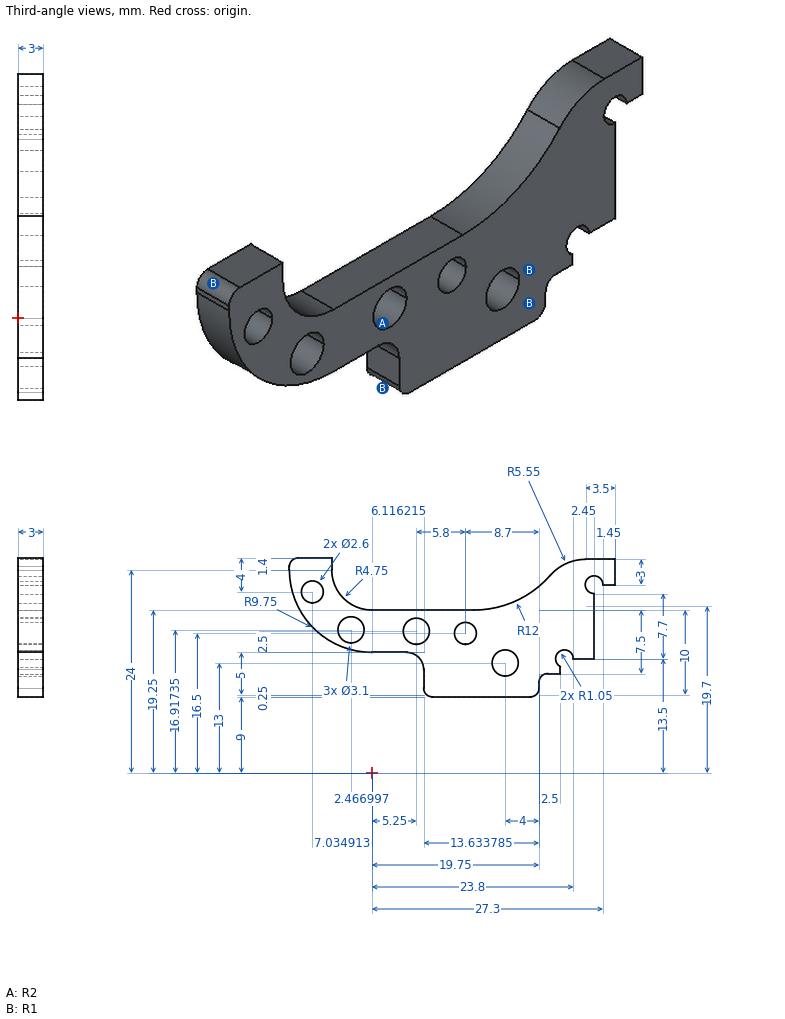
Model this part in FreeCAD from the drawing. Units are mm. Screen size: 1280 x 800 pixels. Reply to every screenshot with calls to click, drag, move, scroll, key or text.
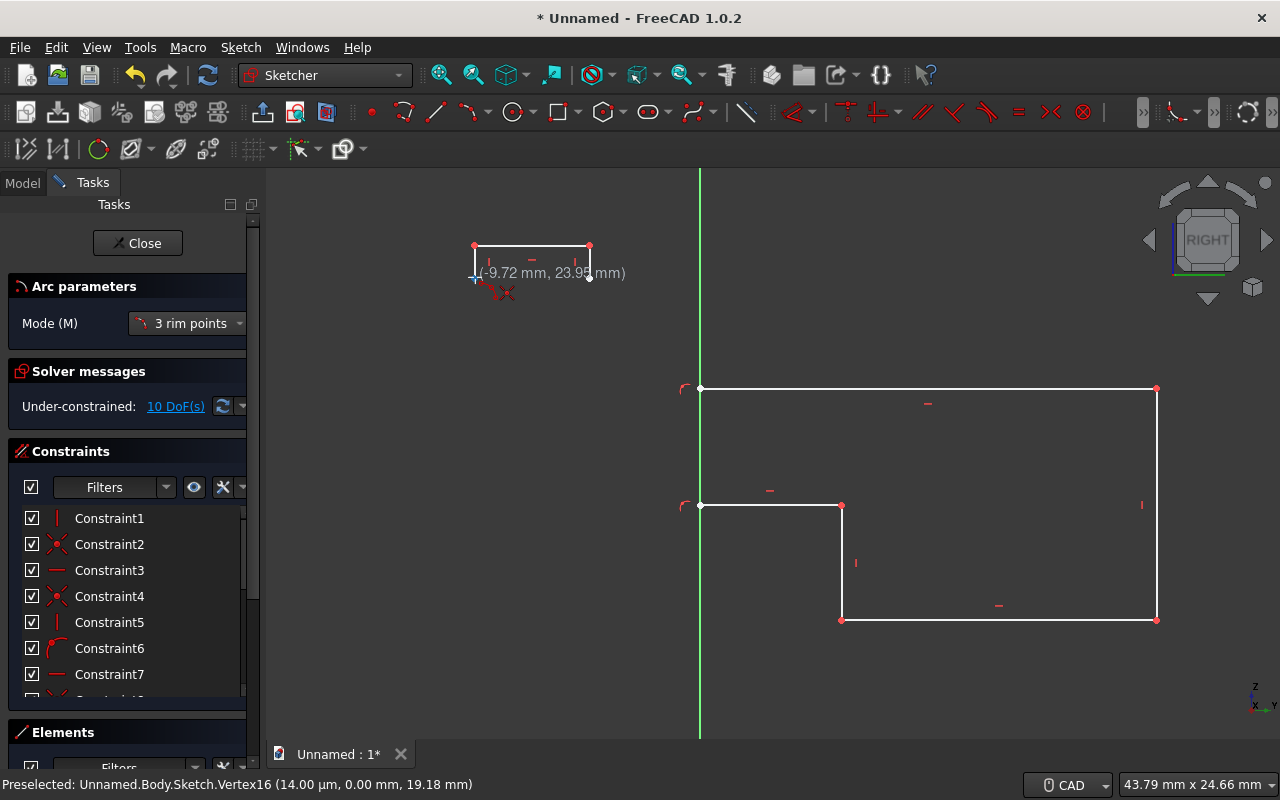
click(475, 278)
click(700, 505)
click(540, 437)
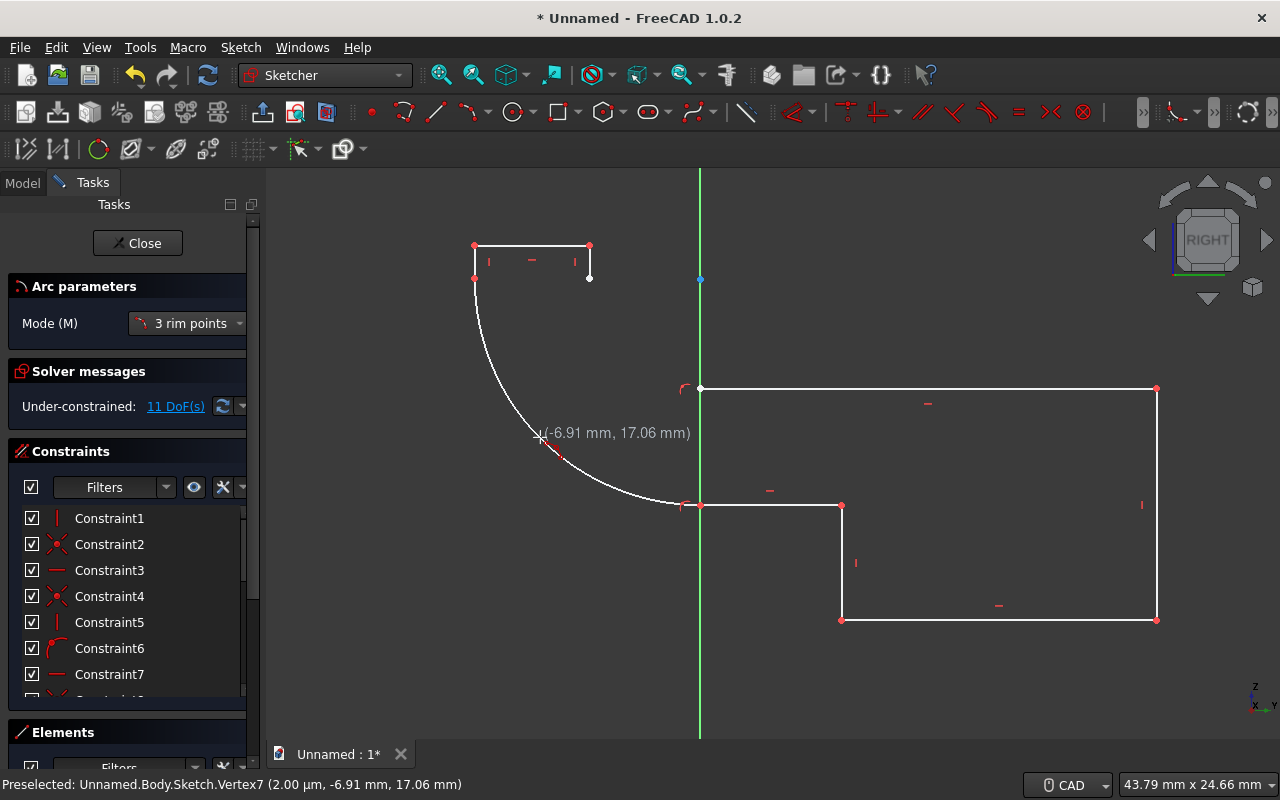
click(700, 389)
click(590, 278)
click(622, 355)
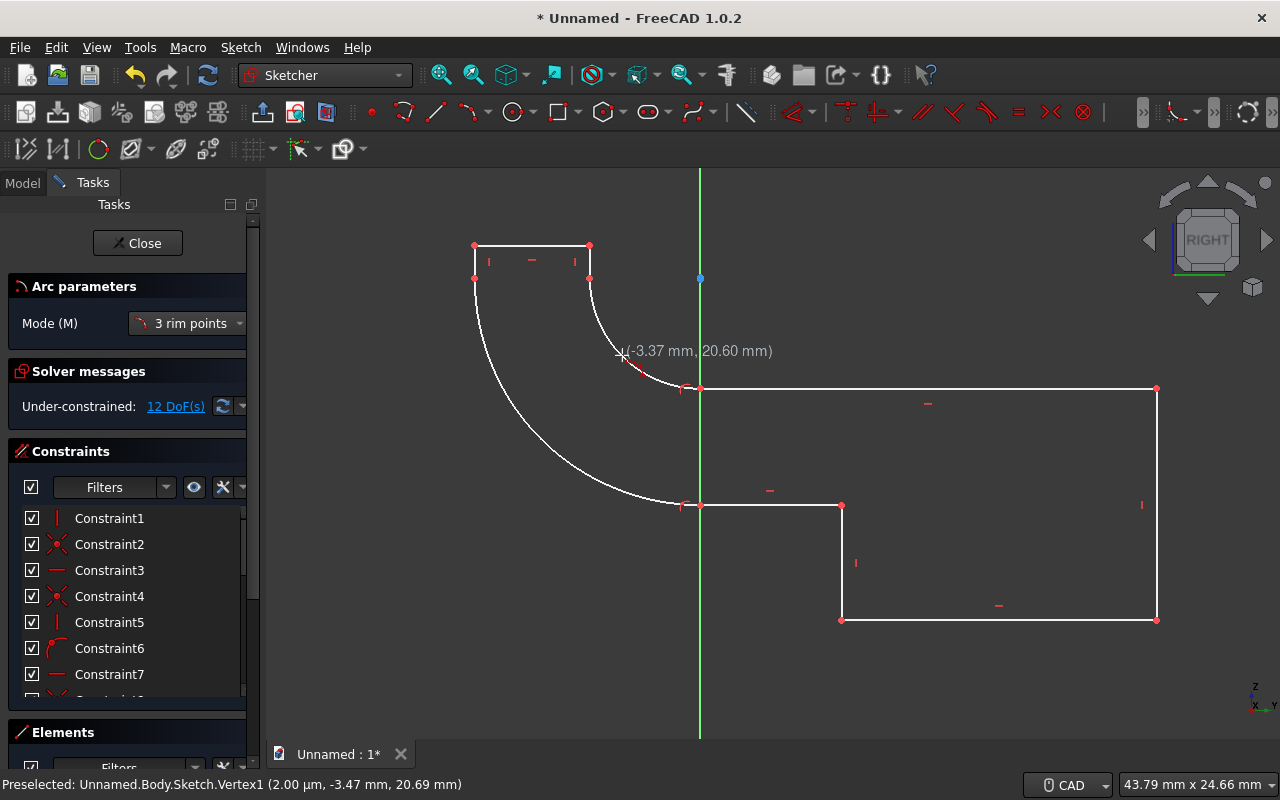
key(g)
key(c)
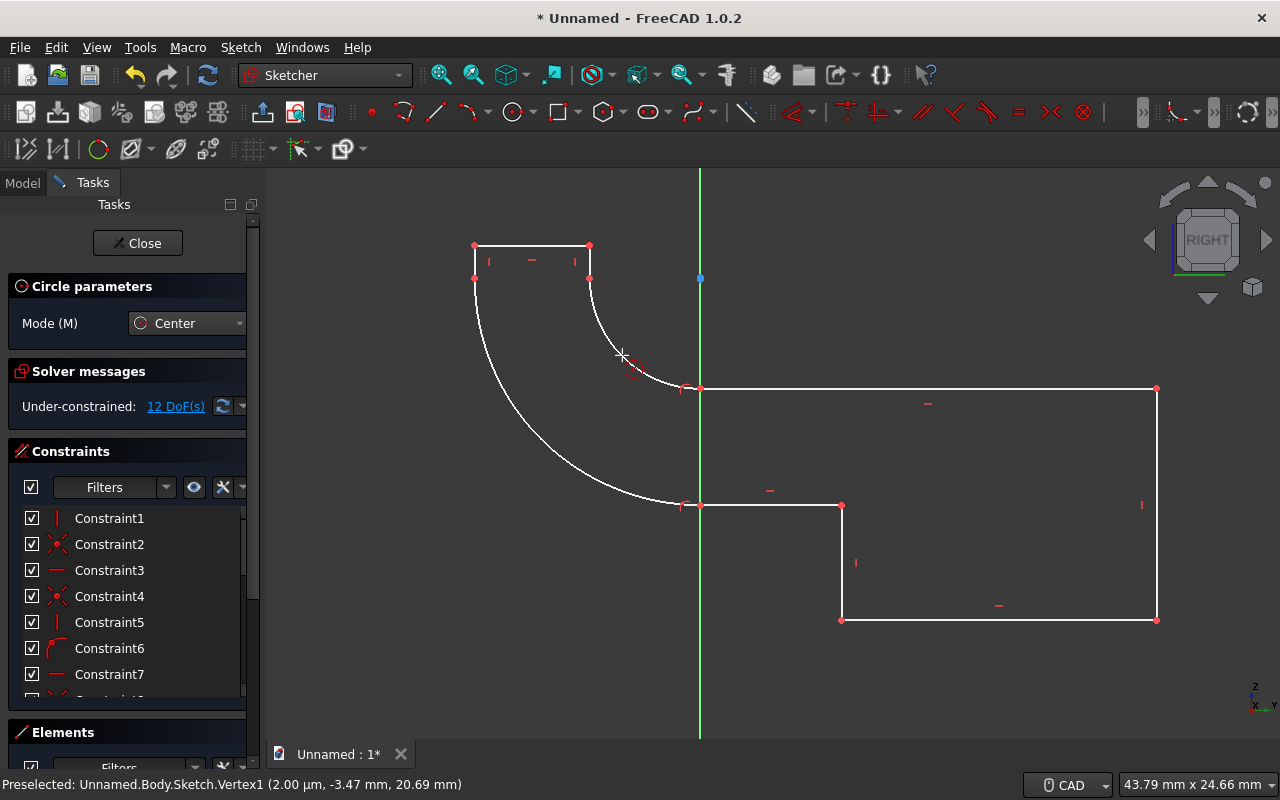
click(537, 337)
click(558, 316)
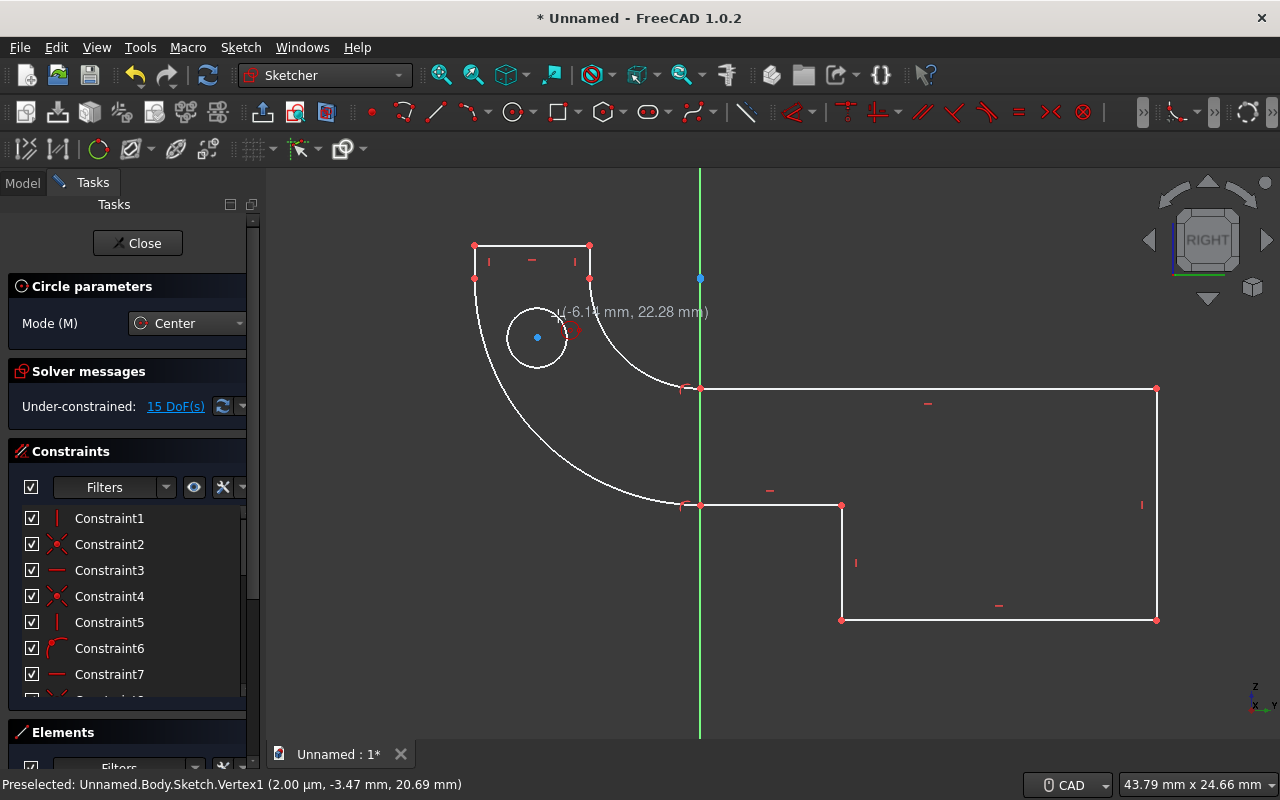
click(643, 441)
click(668, 416)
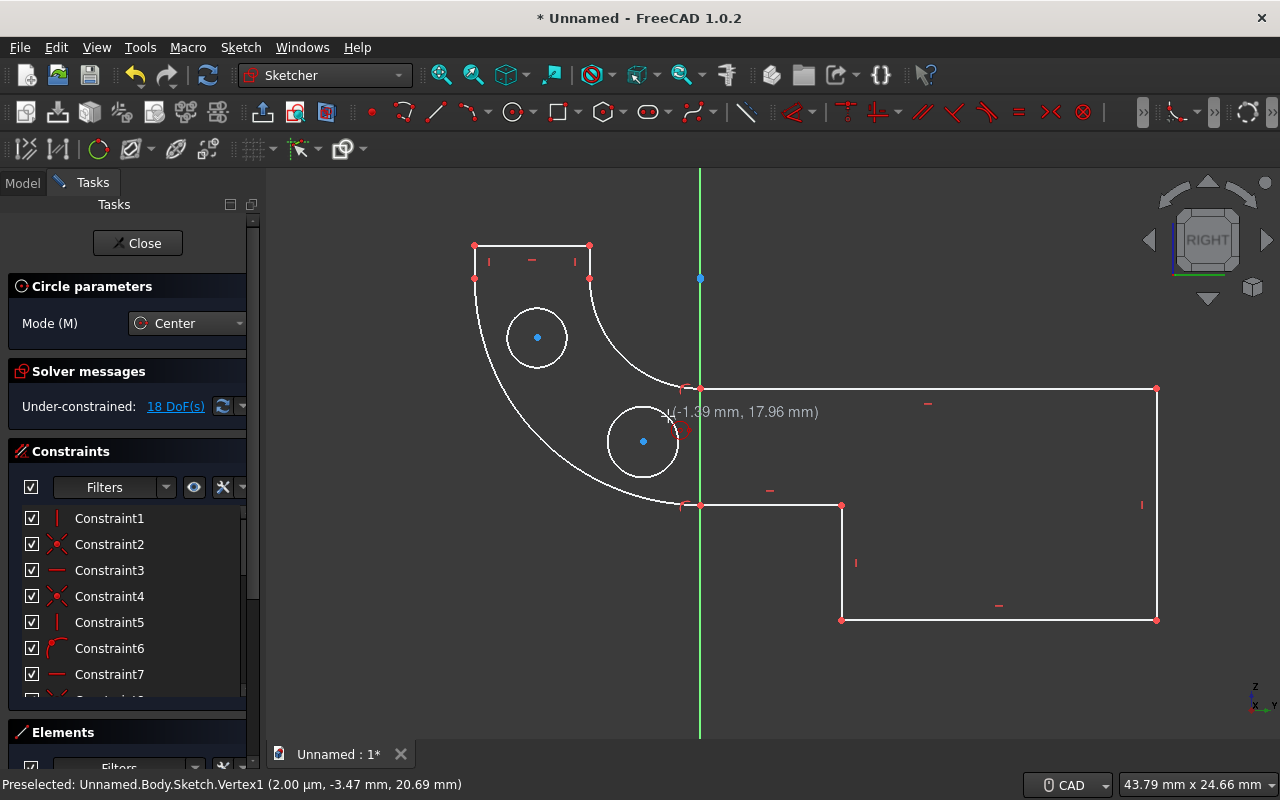
click(822, 445)
click(847, 420)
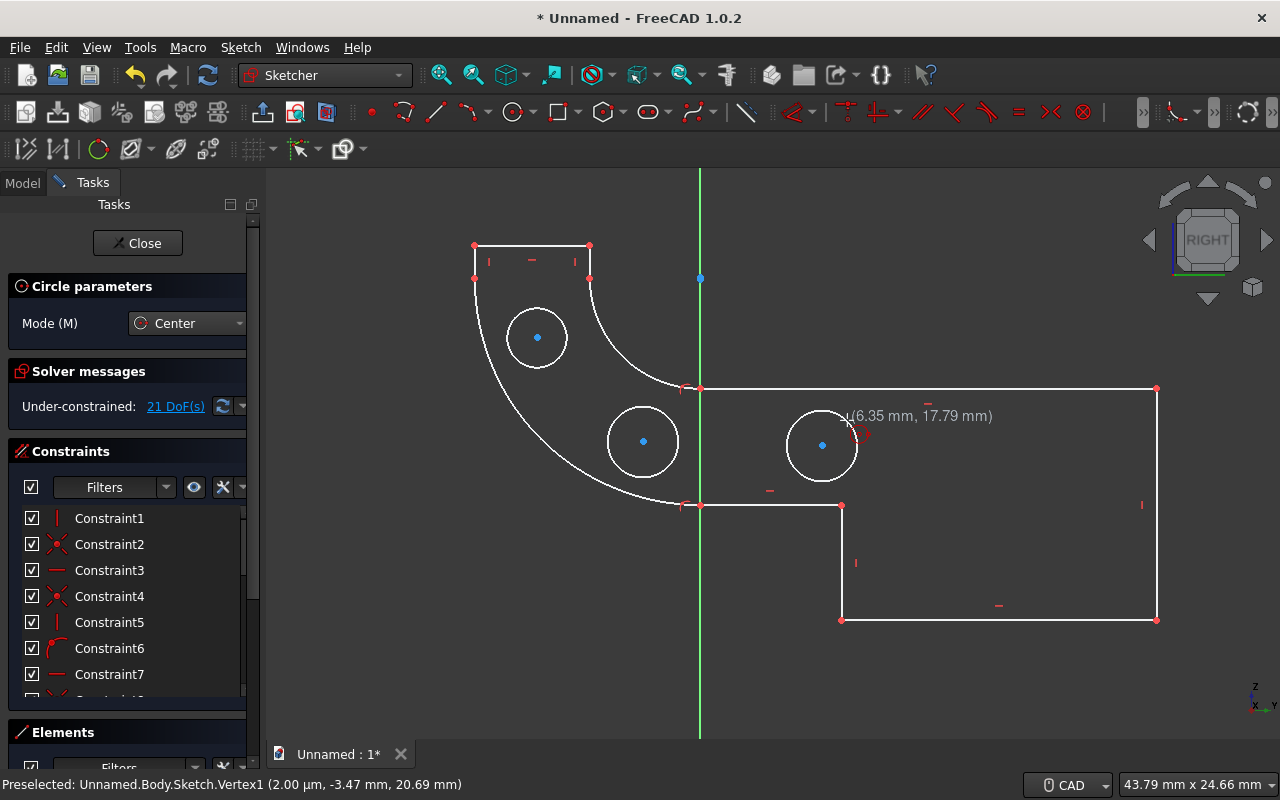
click(956, 451)
click(977, 430)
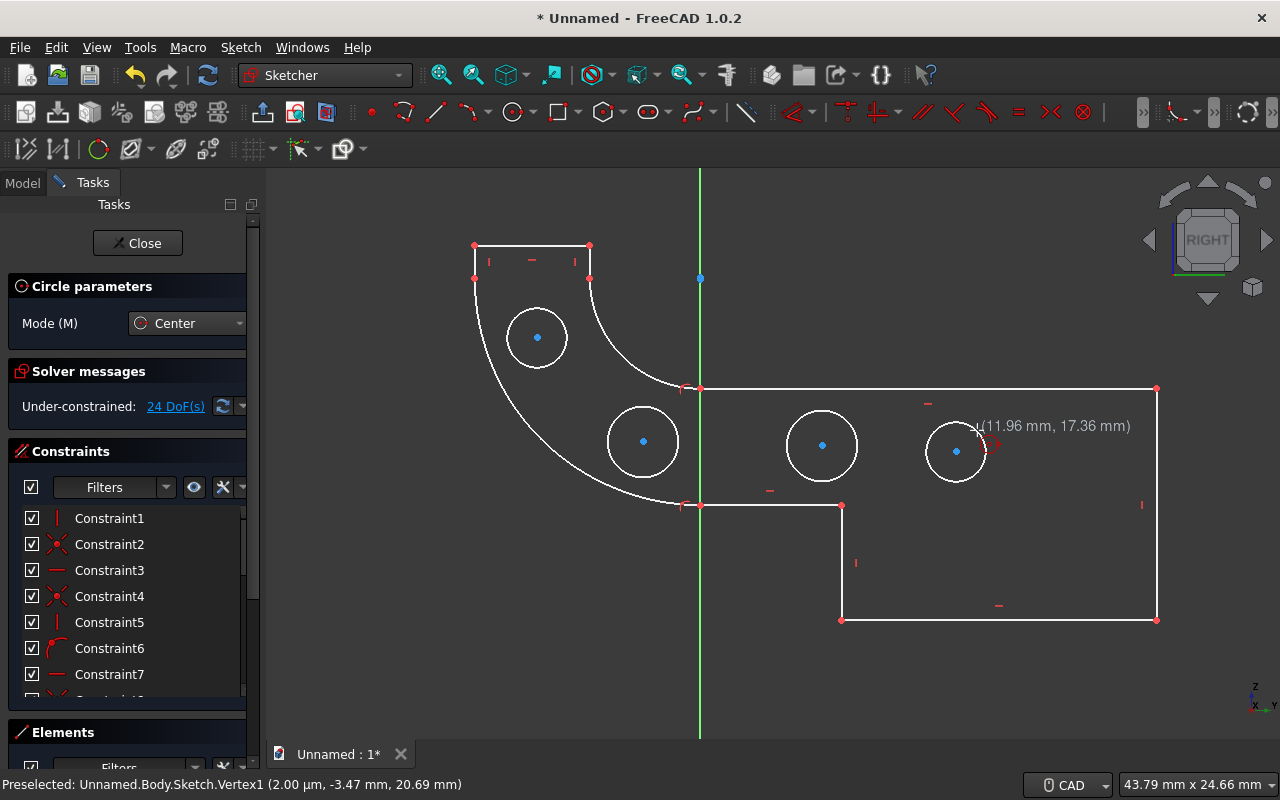
click(1065, 532)
click(1090, 507)
key(Escape)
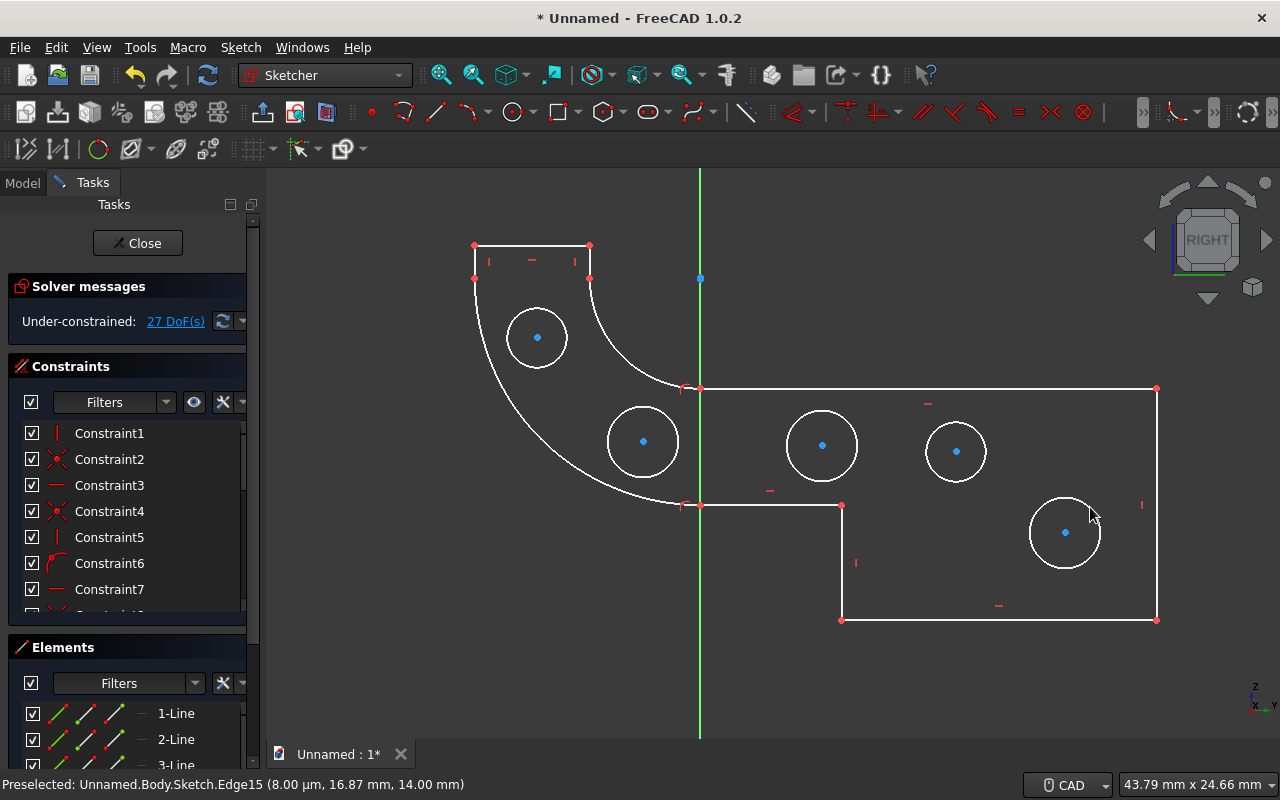
scroll(590, 269, up, 2)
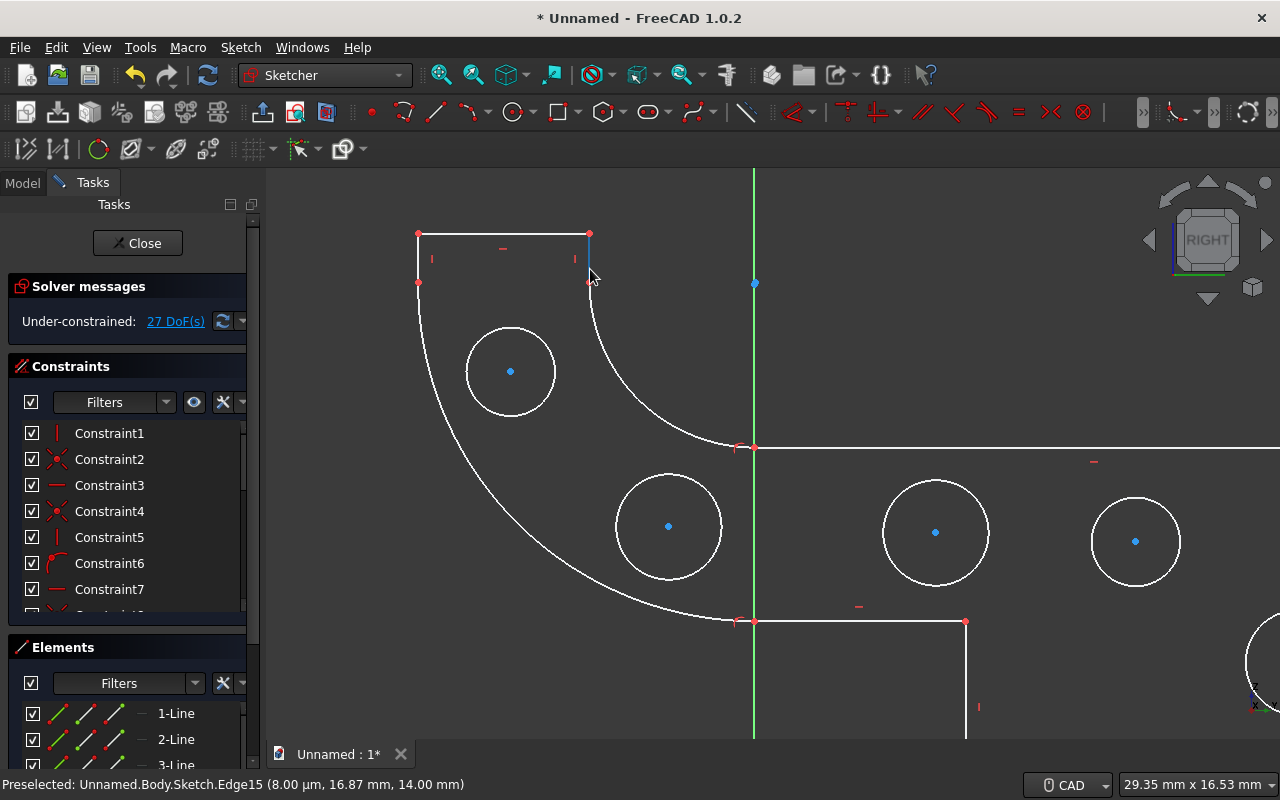
click(589, 268)